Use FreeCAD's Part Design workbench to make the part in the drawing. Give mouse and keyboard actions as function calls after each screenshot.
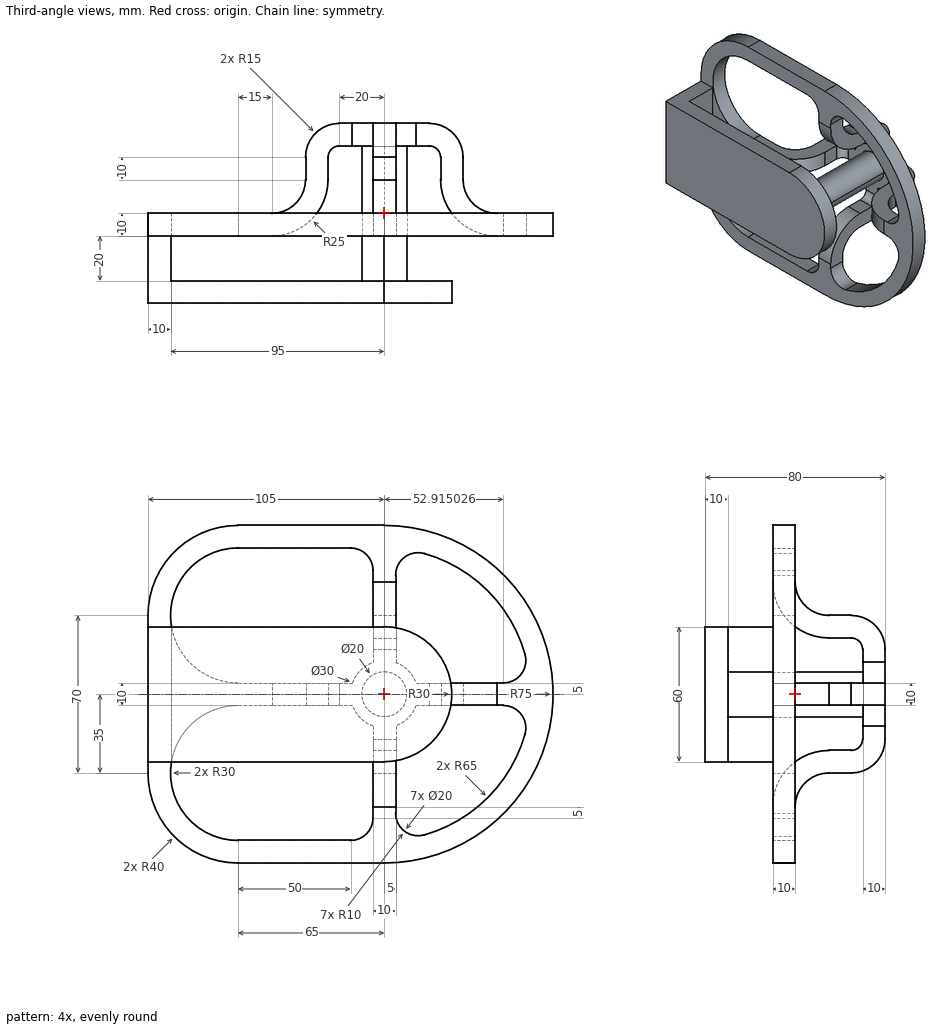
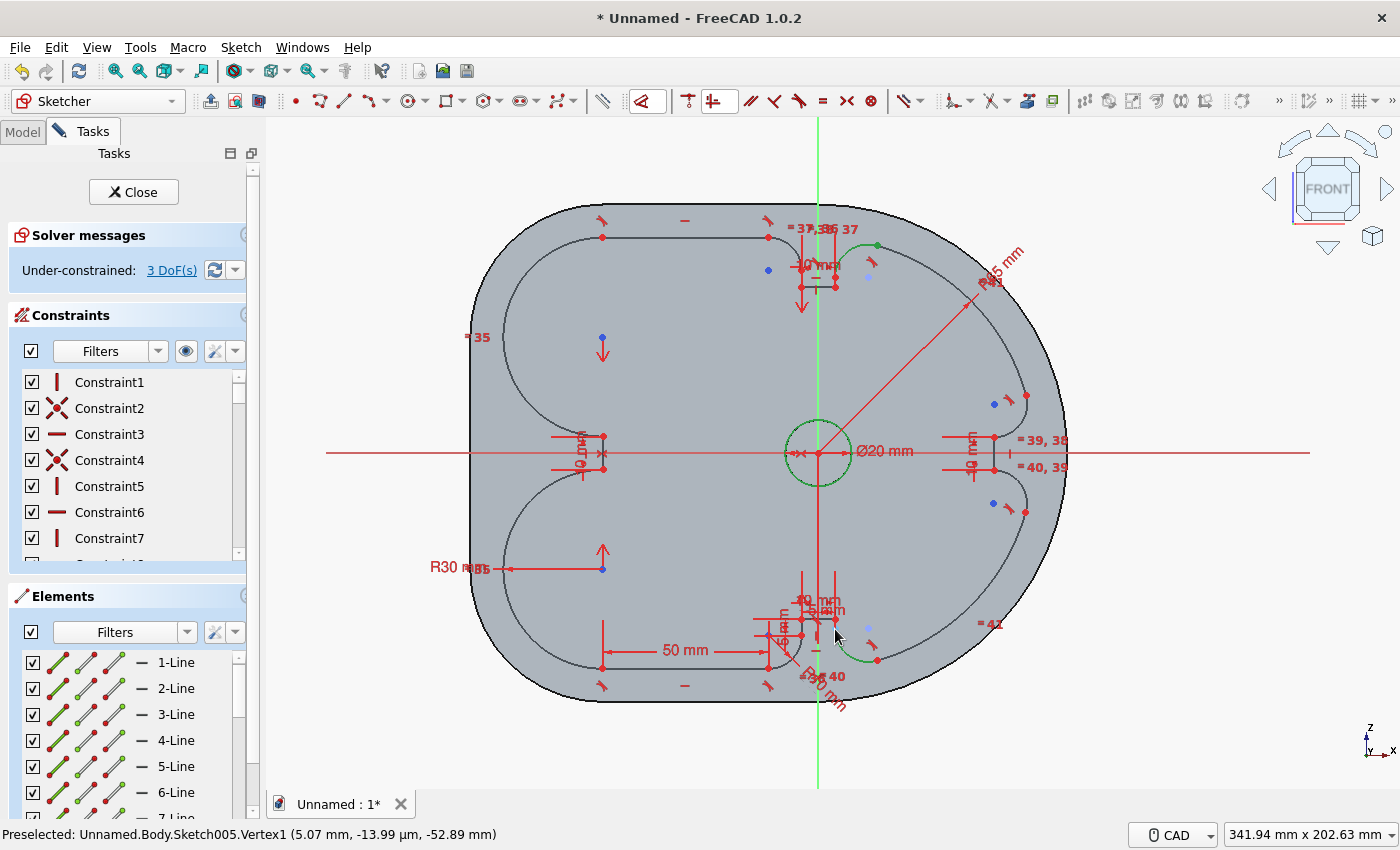
scroll(994, 437, up, 5)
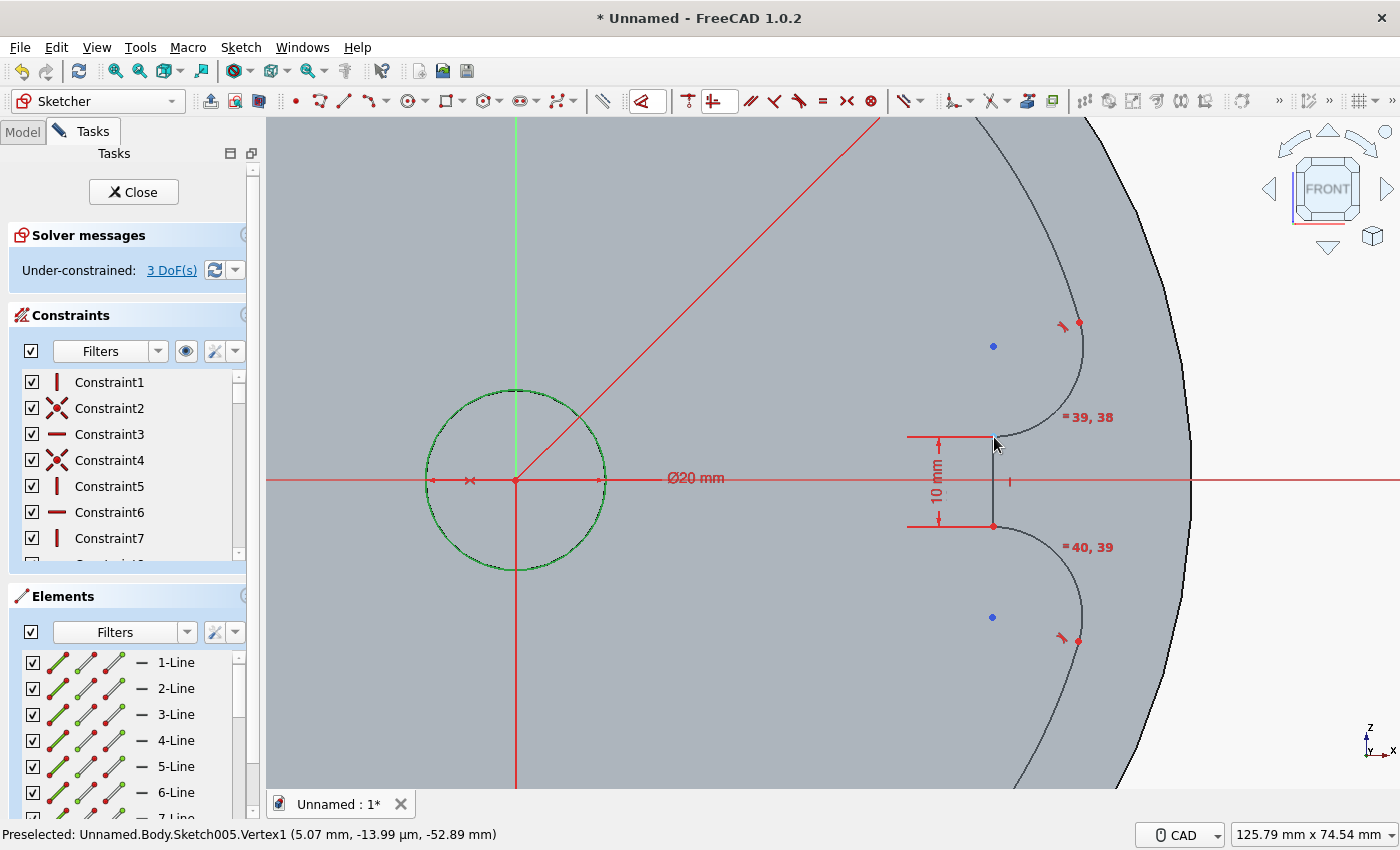
click(993, 437)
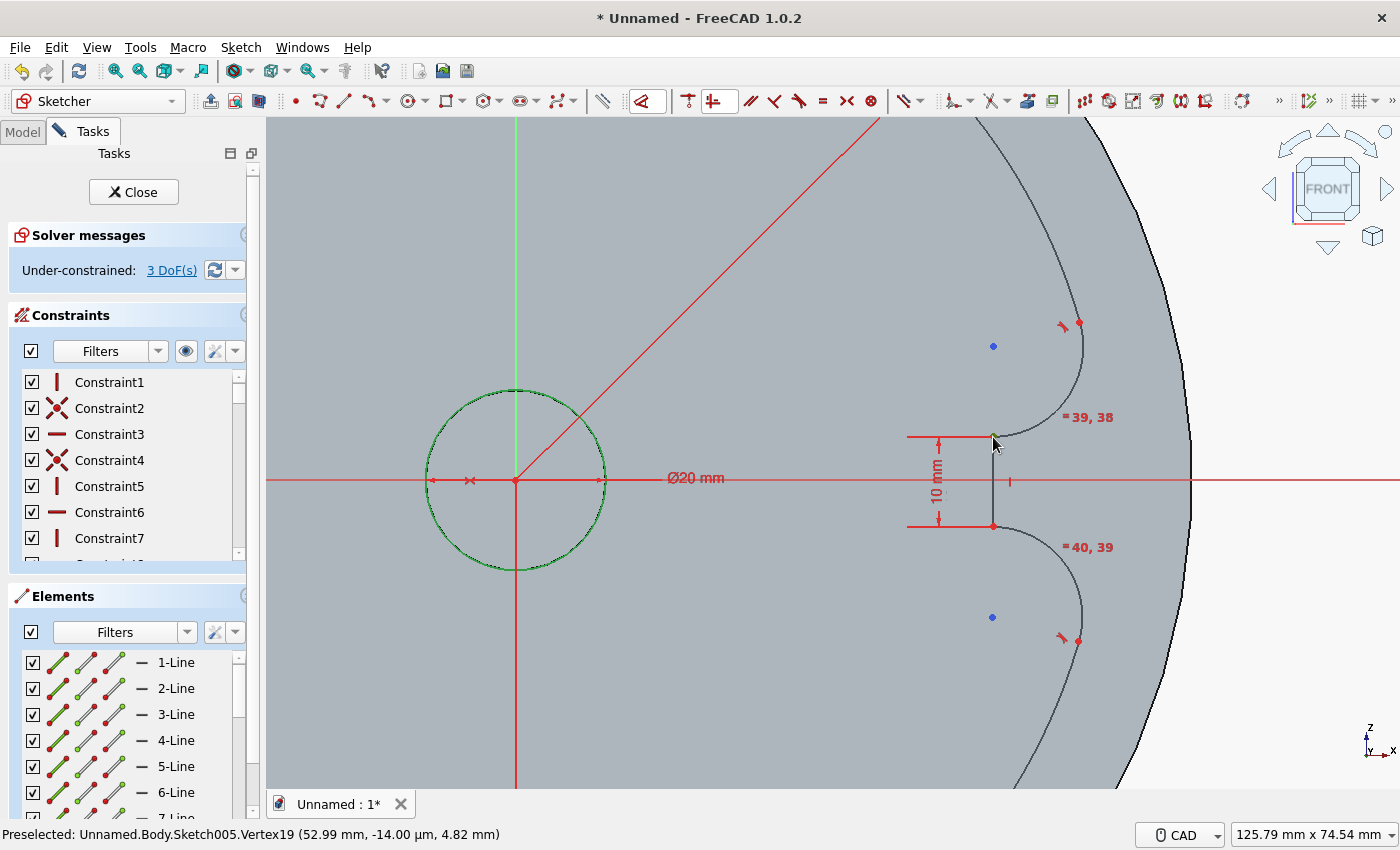
click(660, 102)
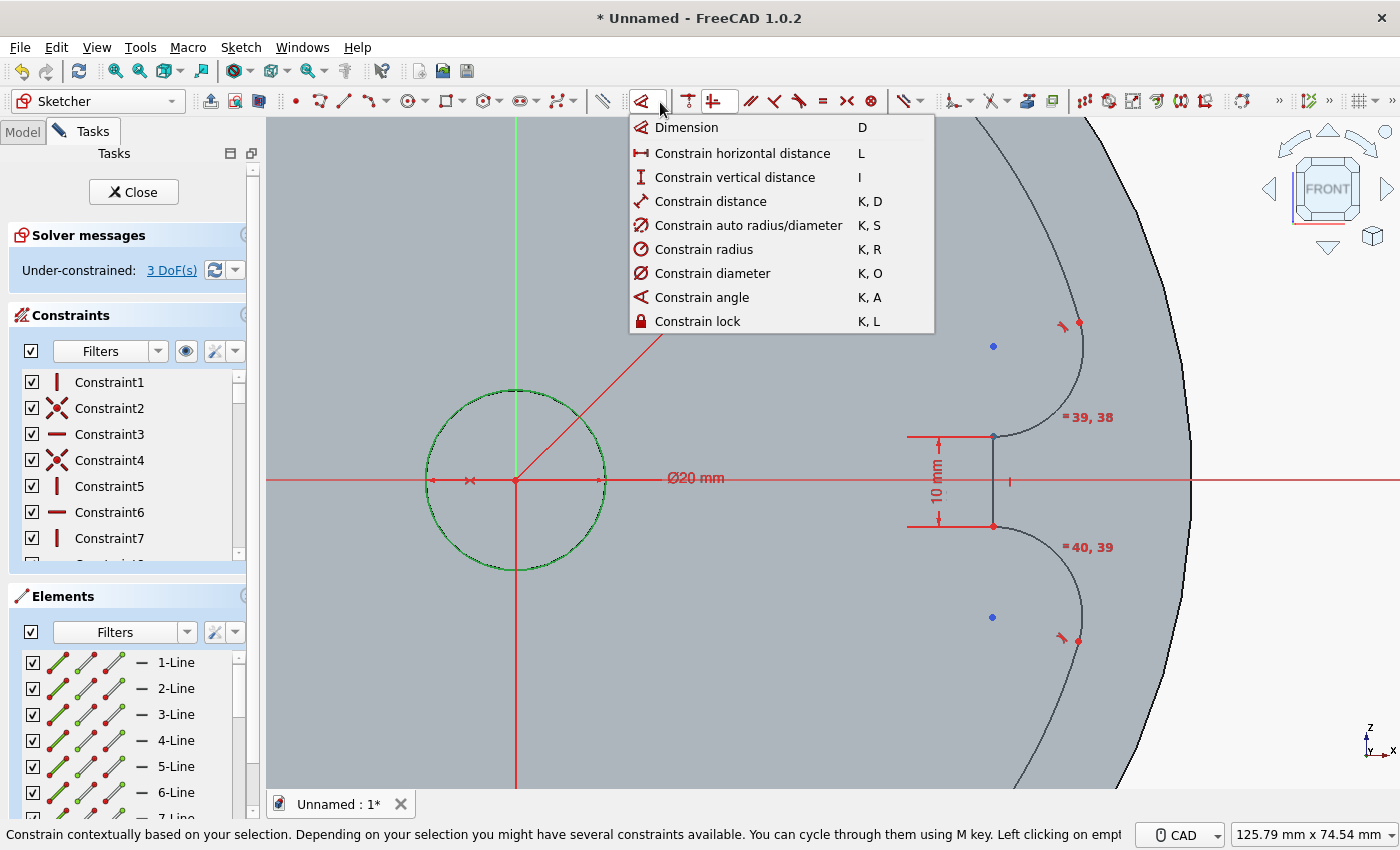
click(782, 177)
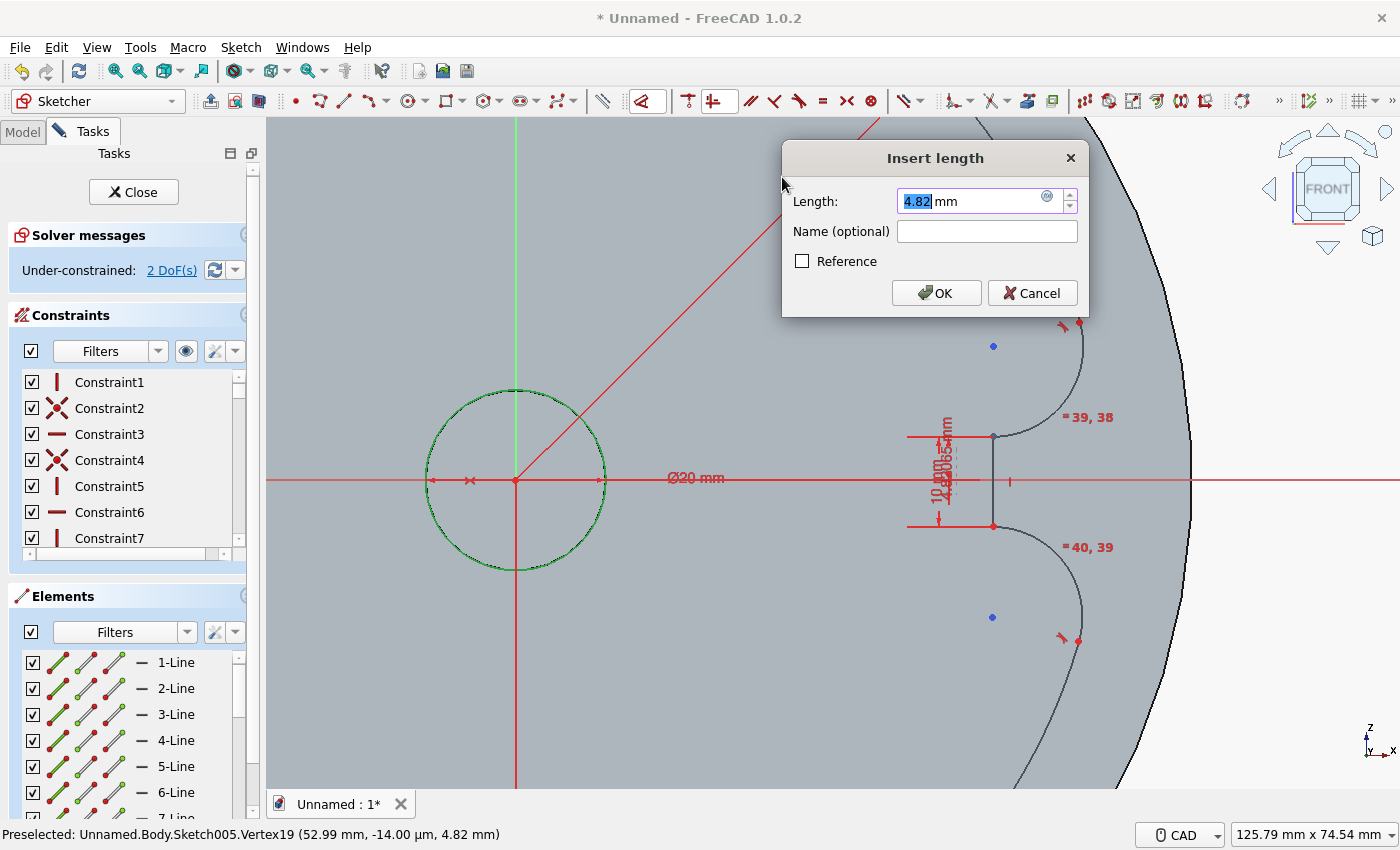
text(5)
key(Return)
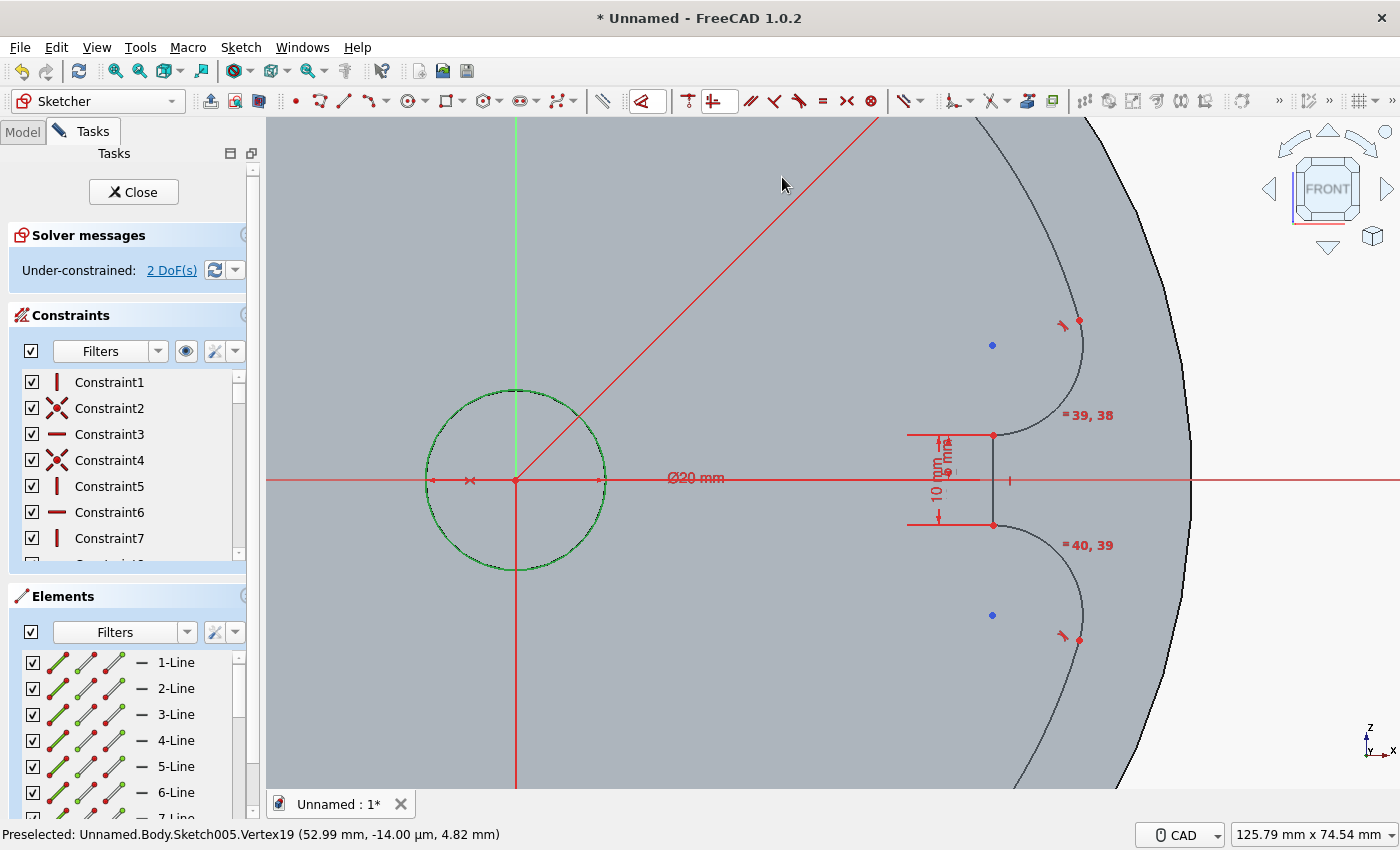
scroll(994, 437, down, 5)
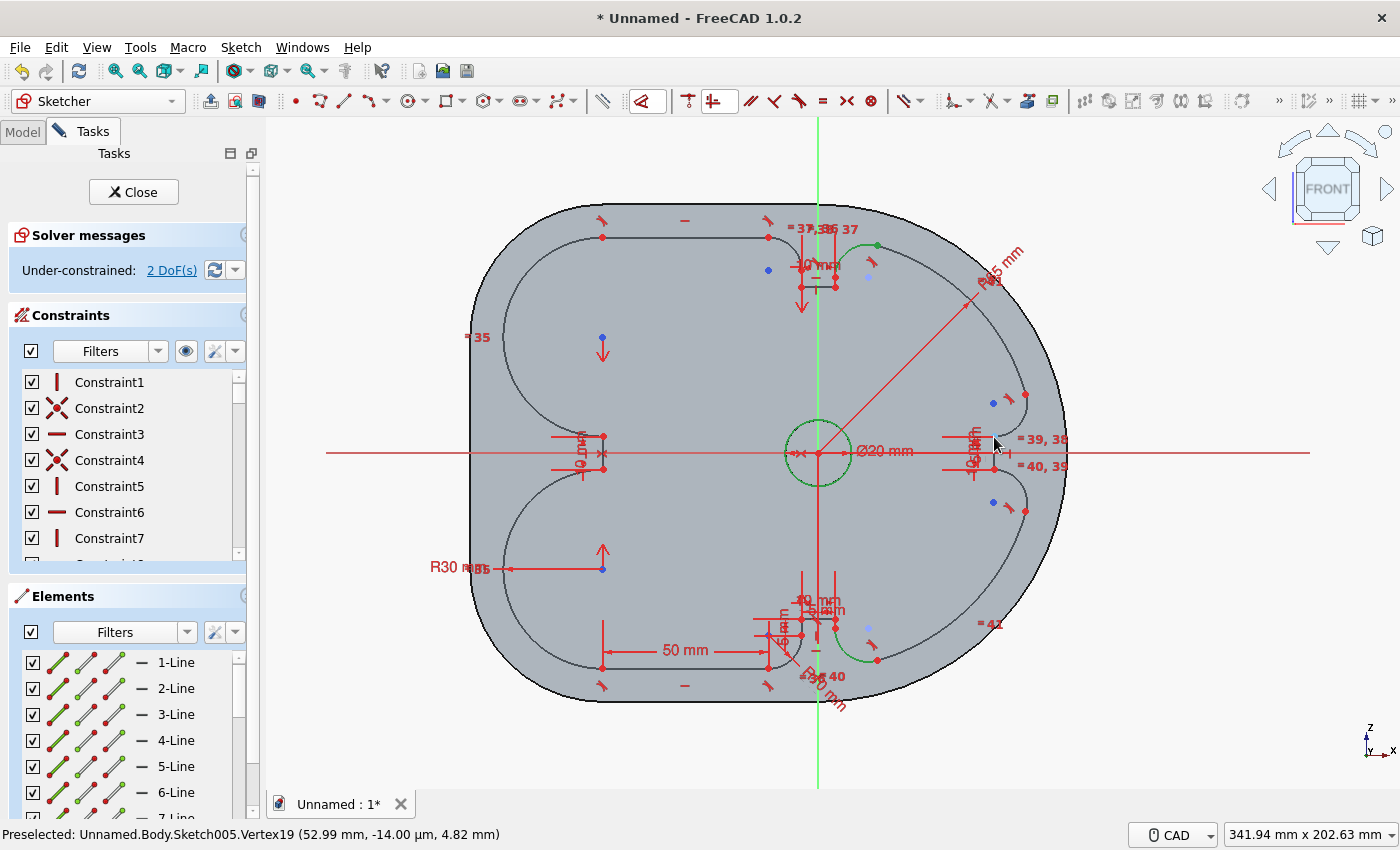
click(603, 470)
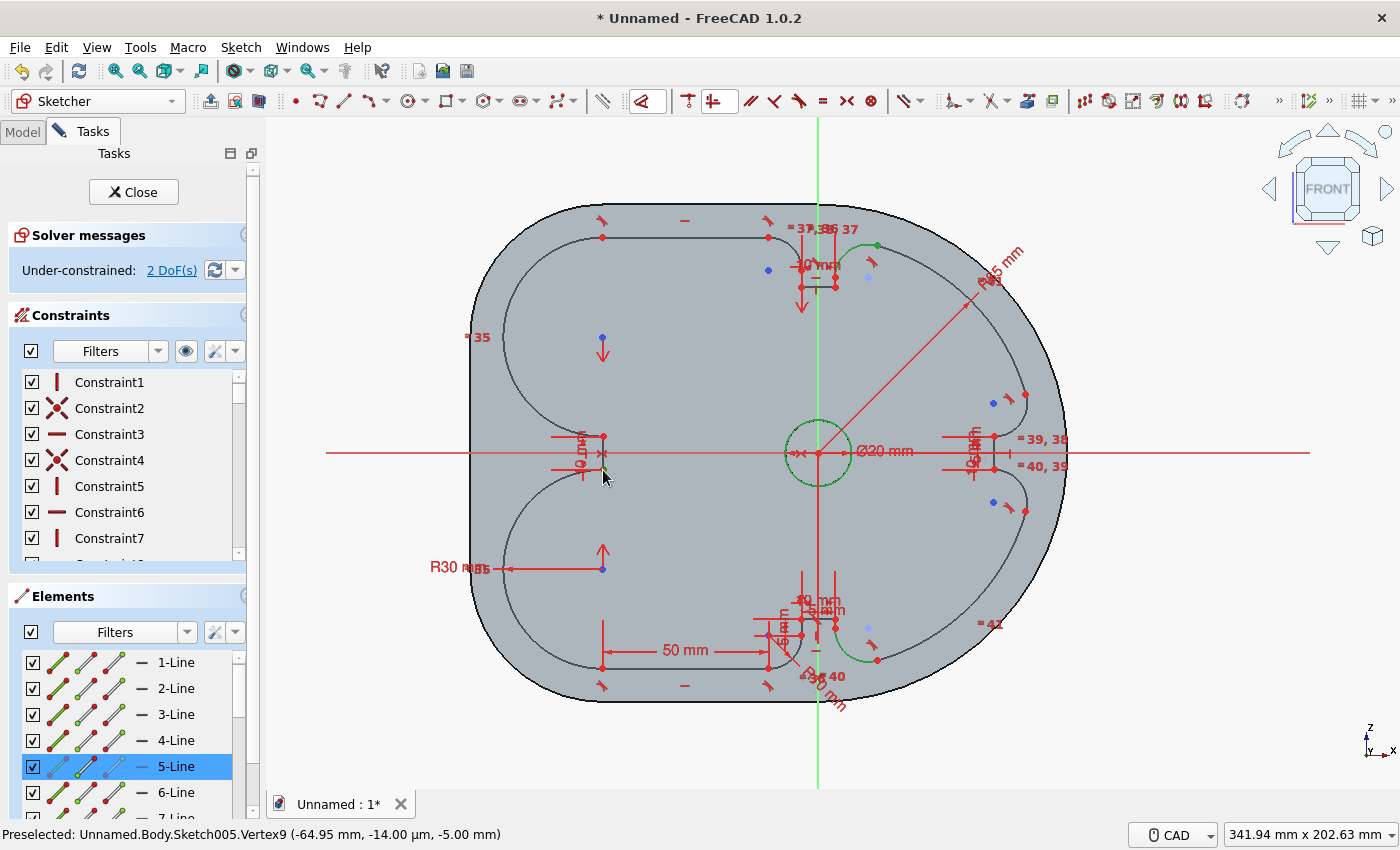
click(660, 102)